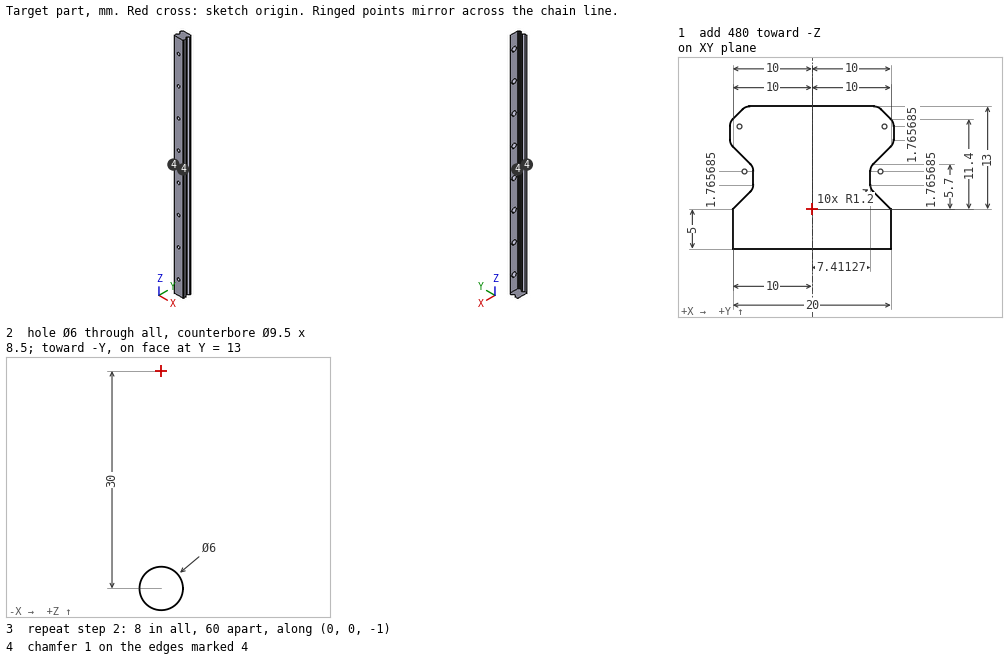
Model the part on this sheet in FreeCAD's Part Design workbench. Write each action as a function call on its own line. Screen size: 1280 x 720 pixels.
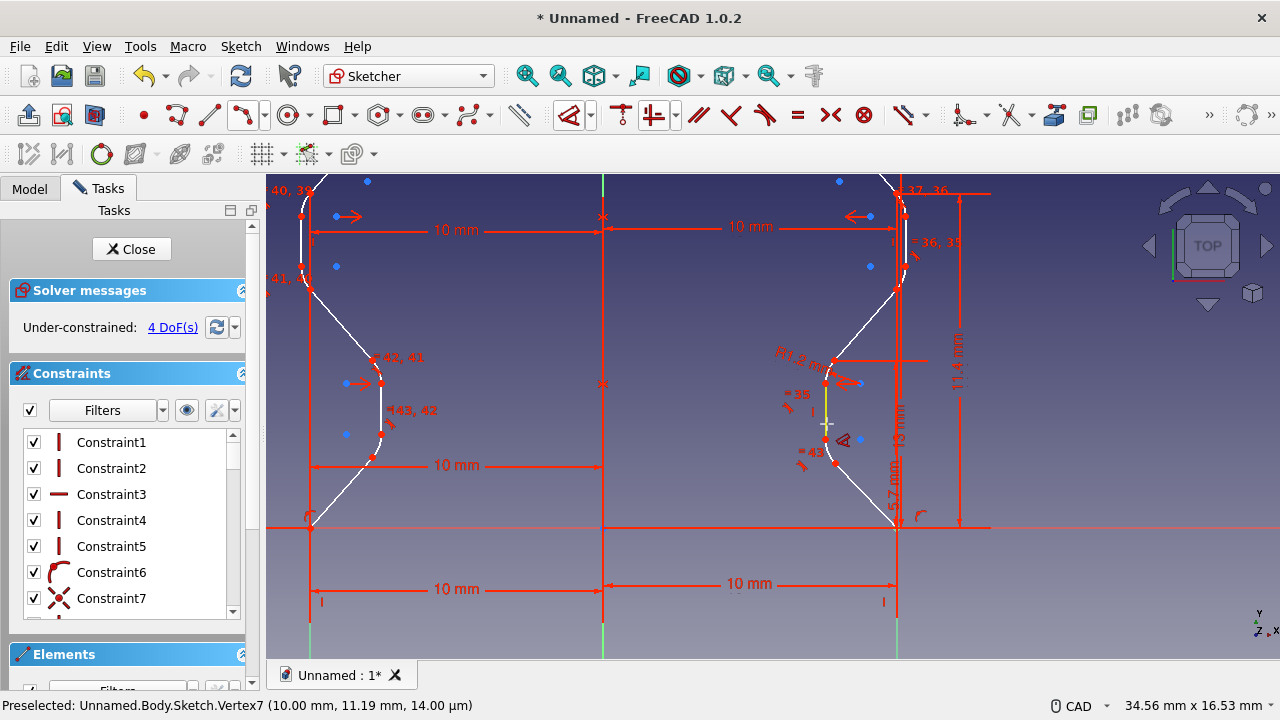
click(826, 423)
click(860, 399)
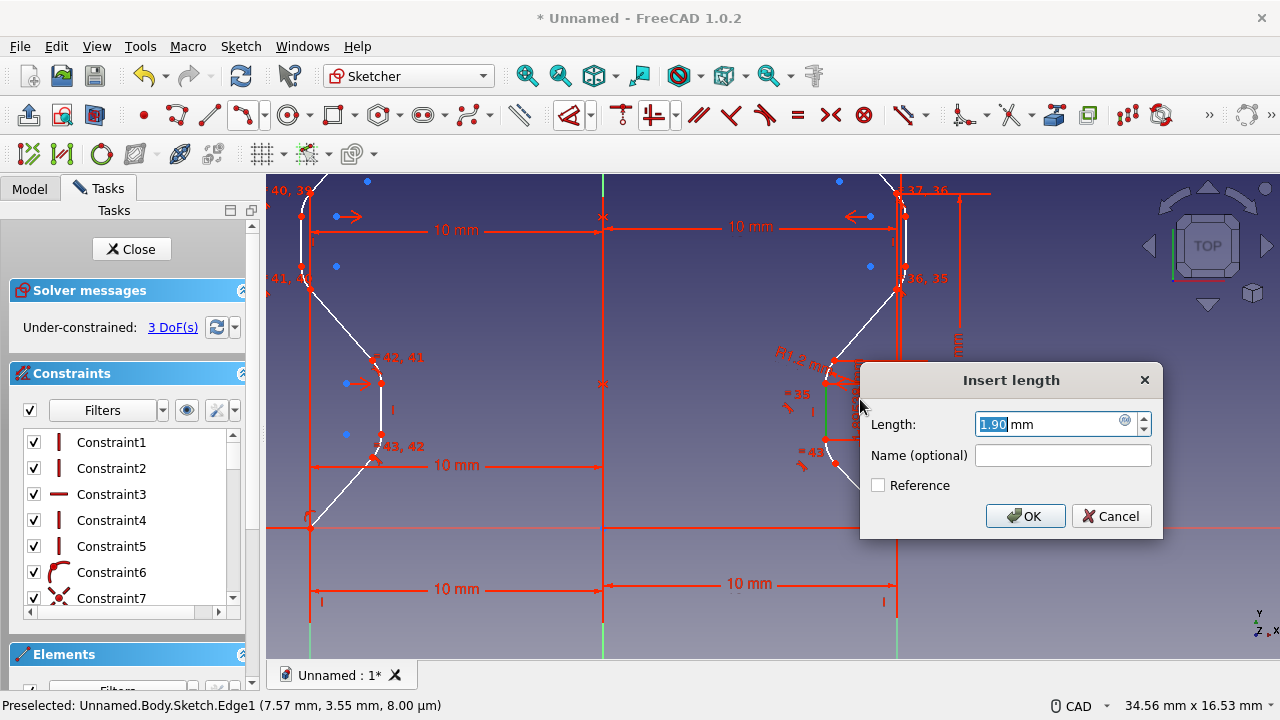
text(1.765685)
key(Return)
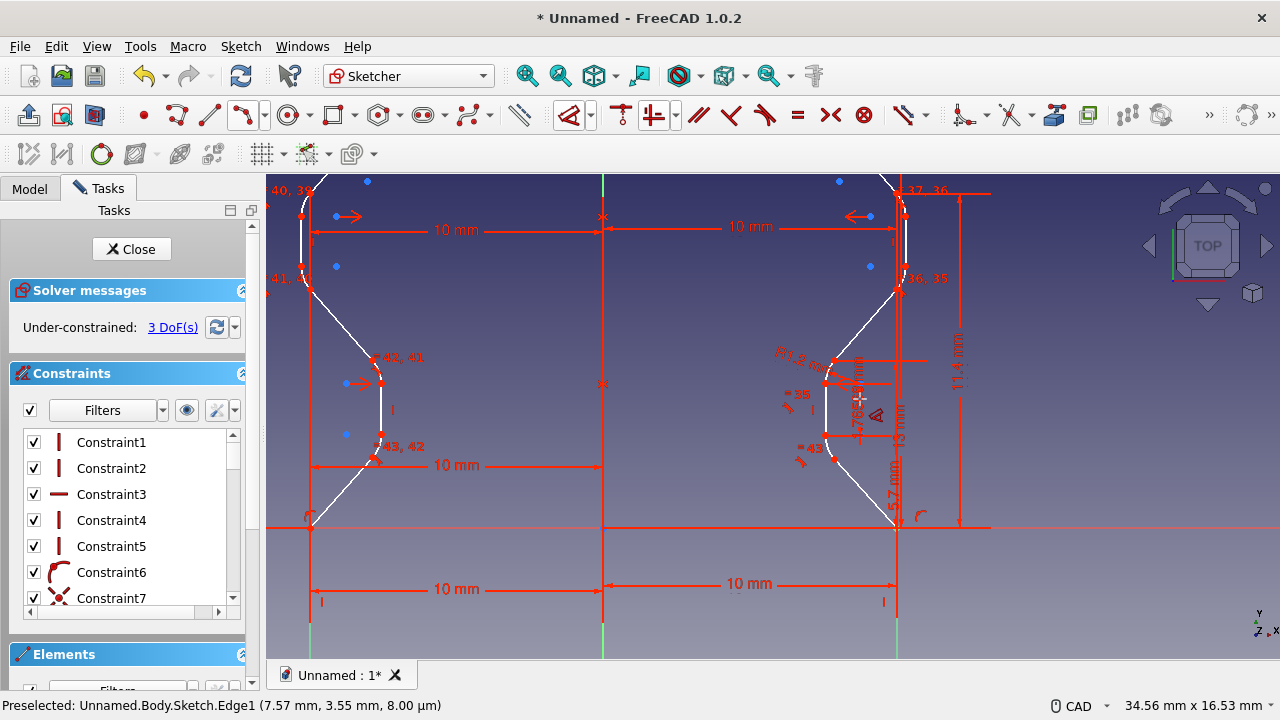
click(906, 251)
click(940, 241)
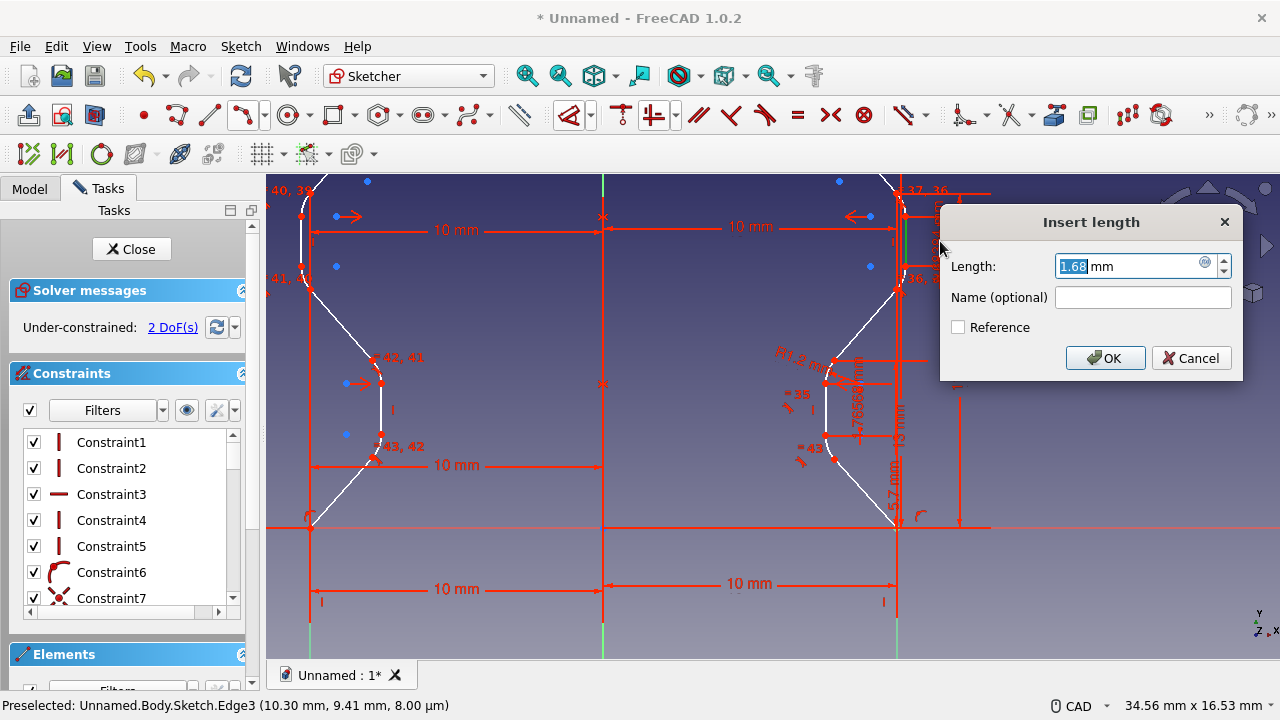
text(1.765685)
key(Return)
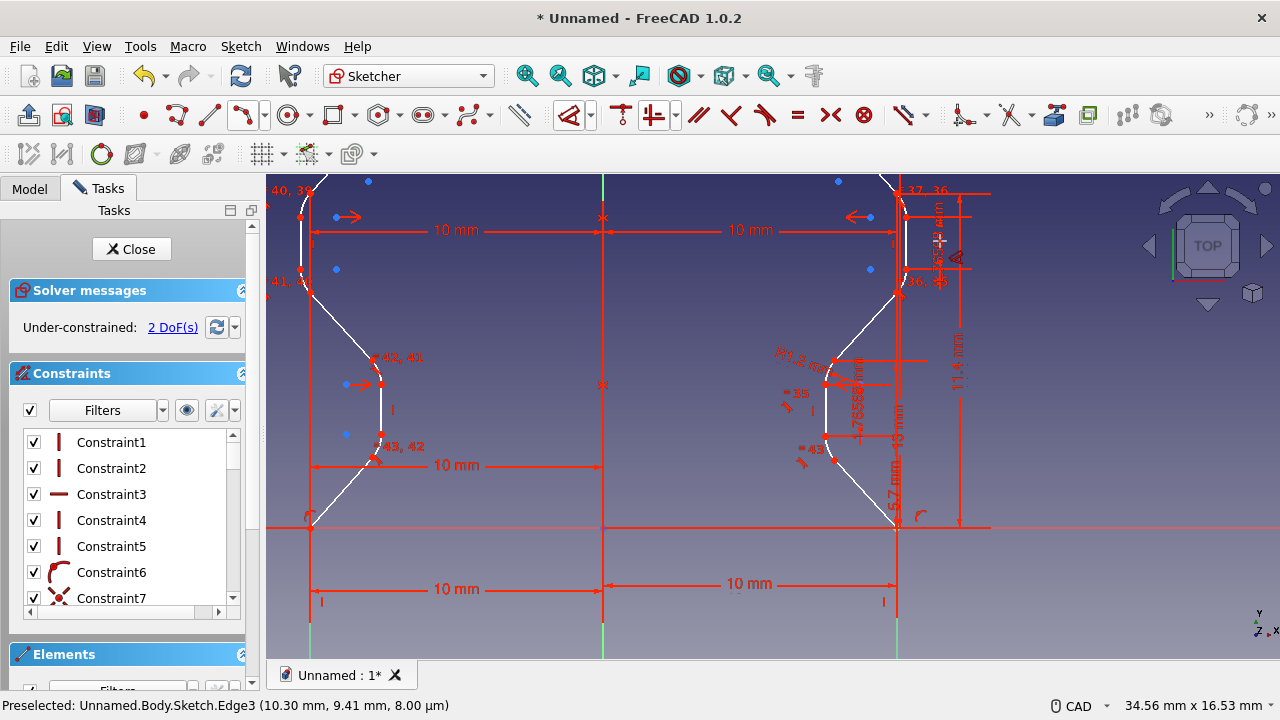
click(381, 400)
click(347, 410)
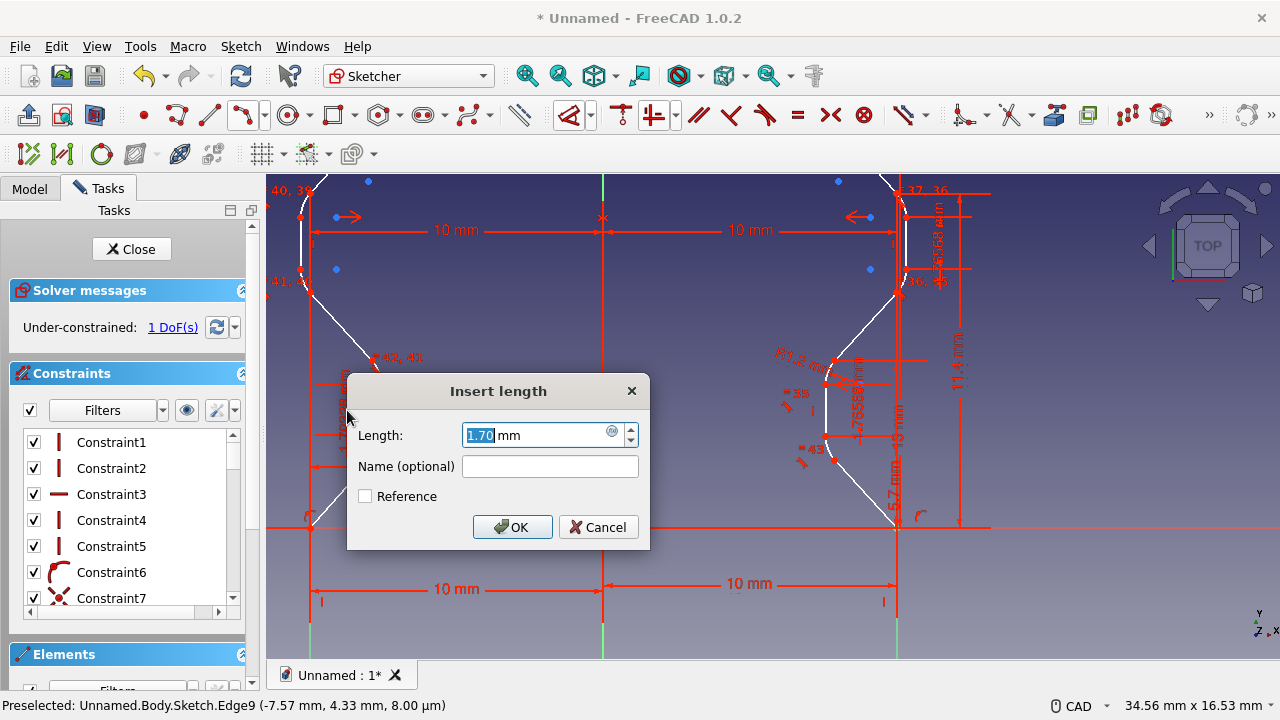
text(1.765685)
key(Return)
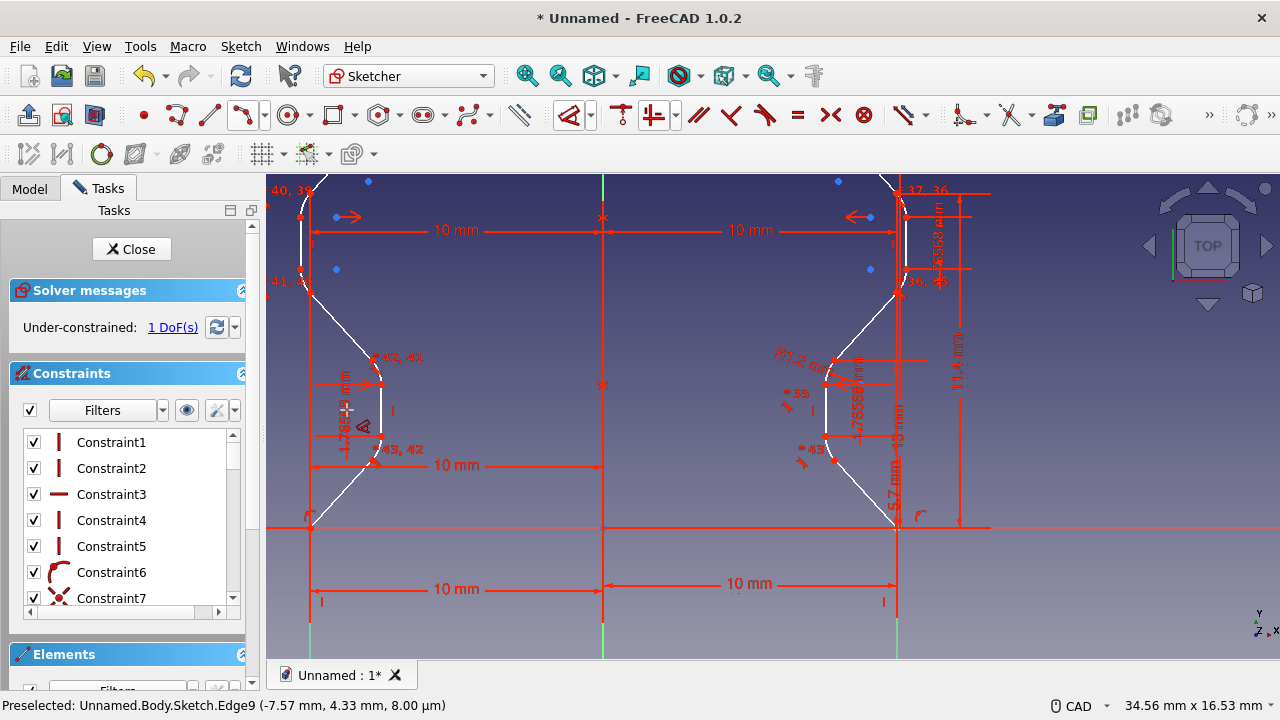
click(826, 436)
click(715, 562)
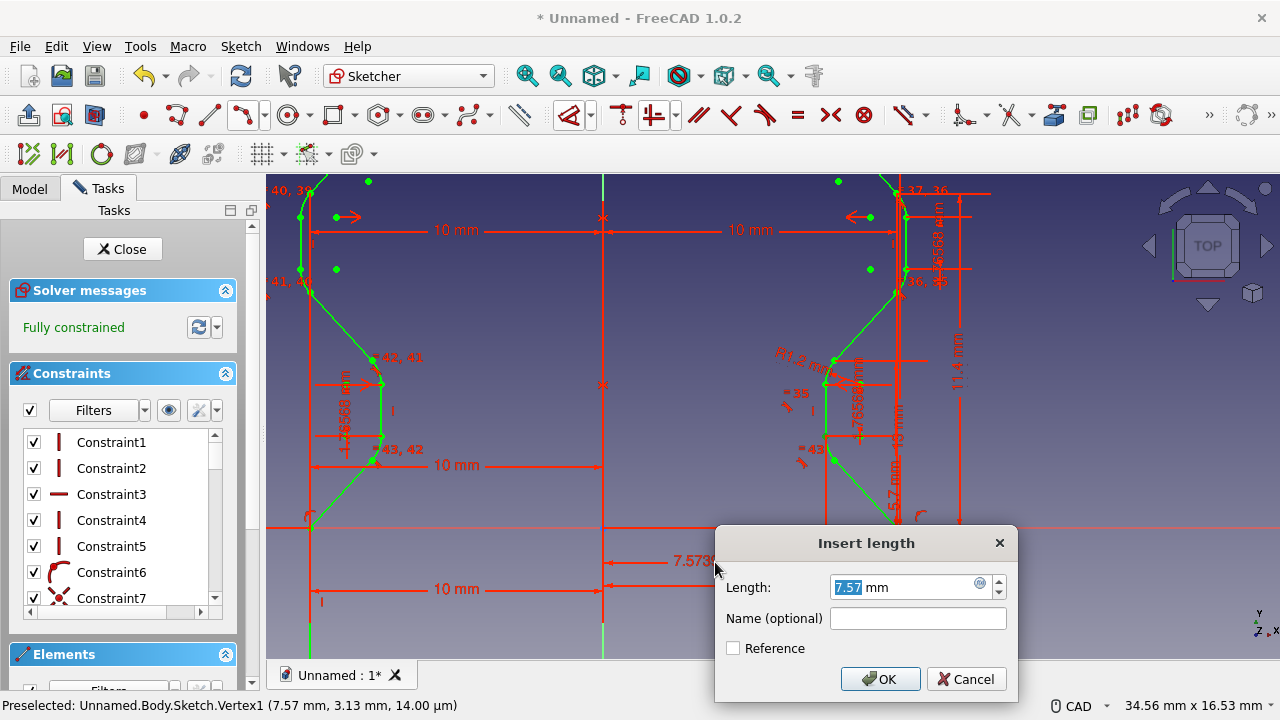
text(7.41127)
key(Return)
key(Escape)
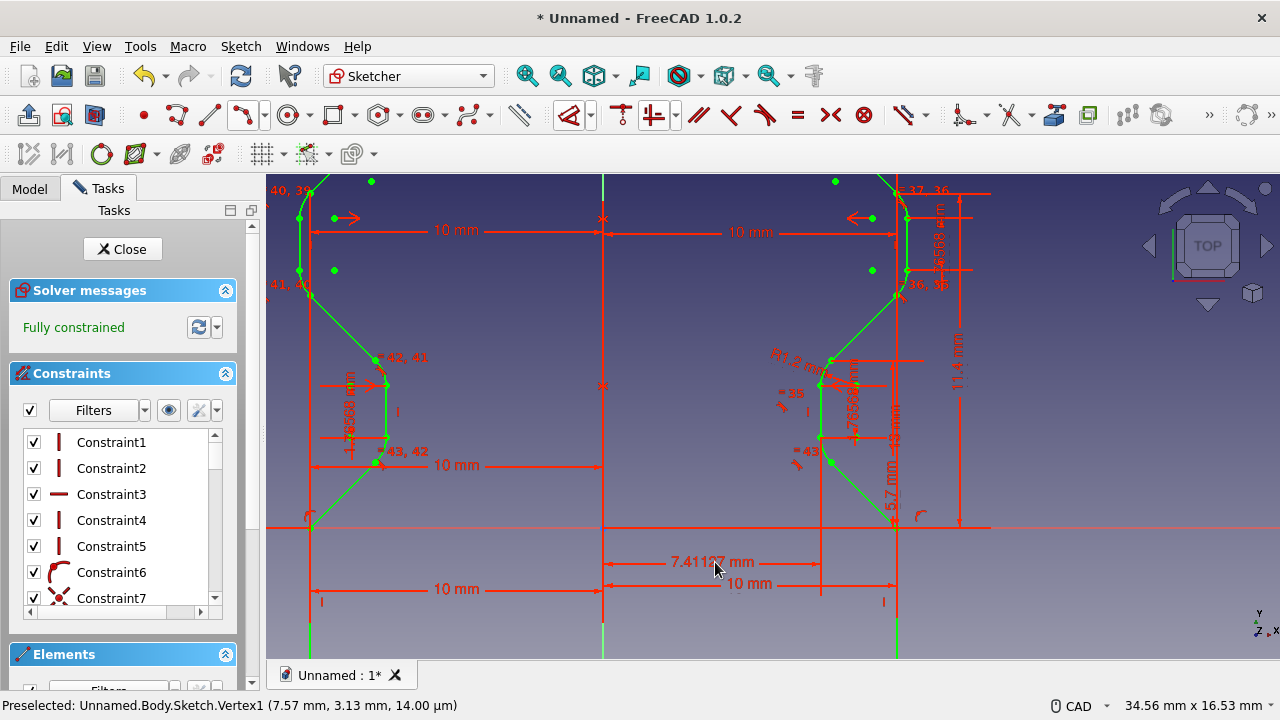
click(123, 249)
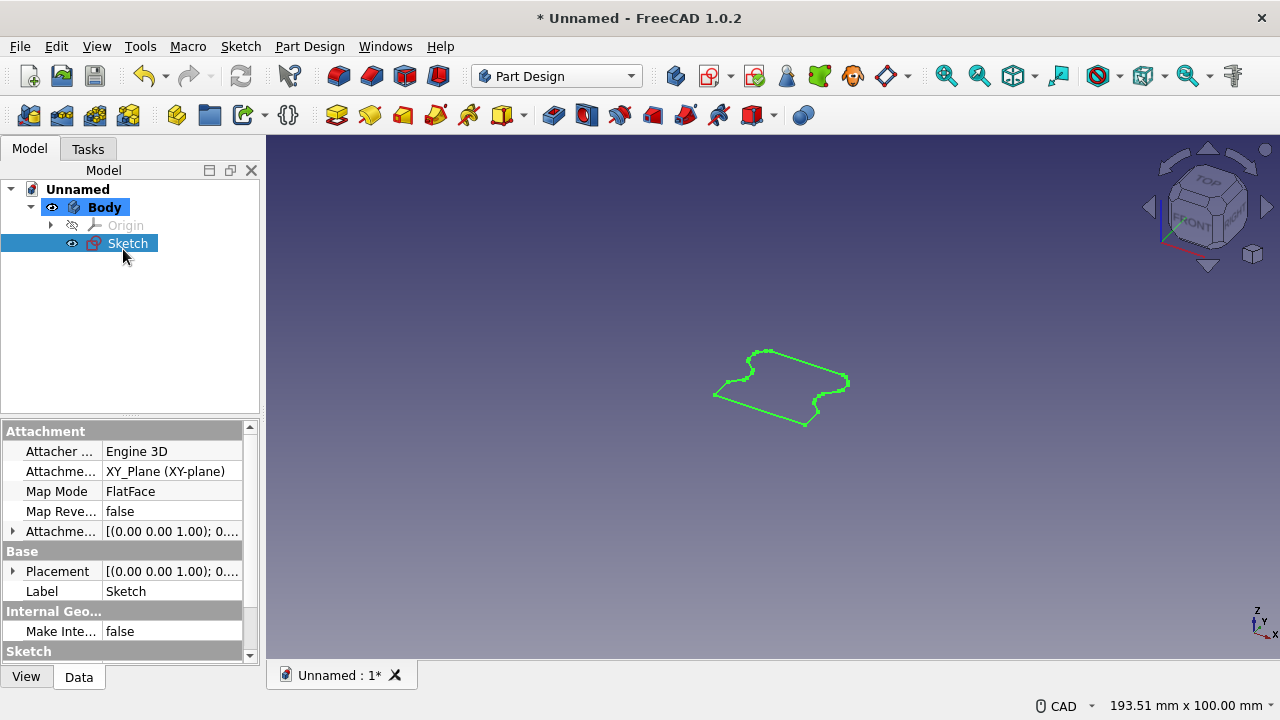
click(337, 116)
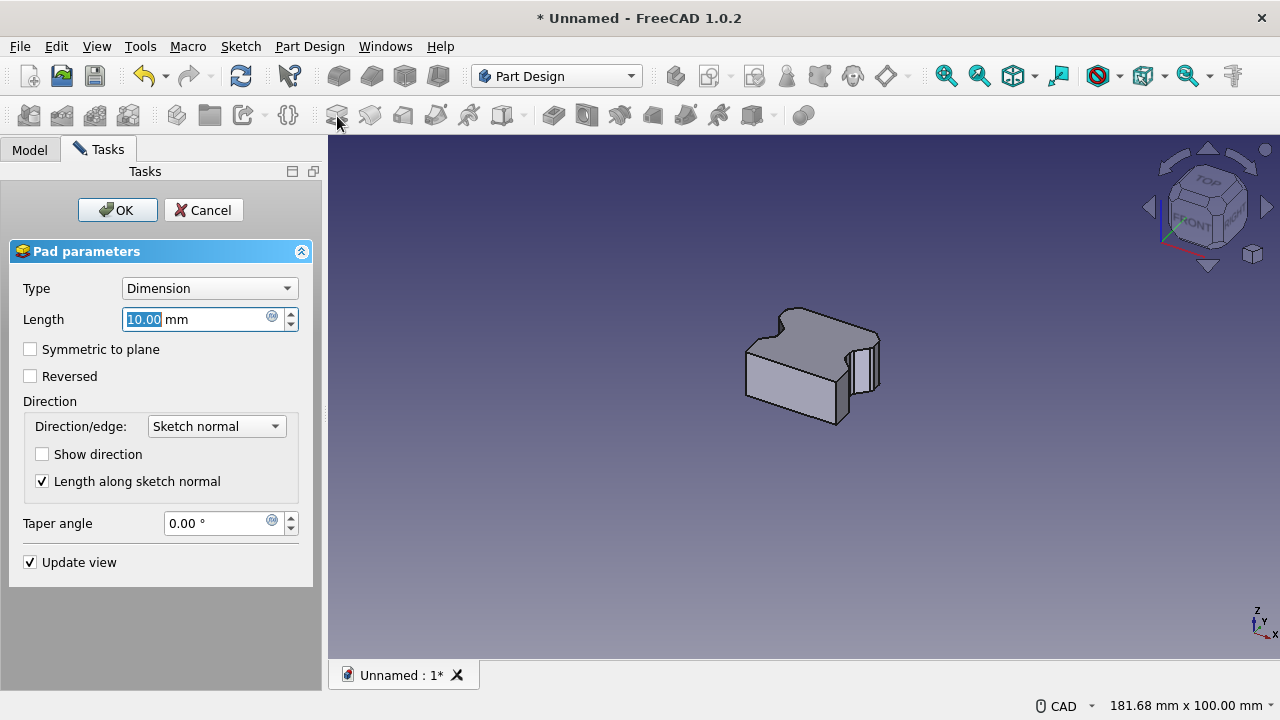
text(480)
key(Tab)